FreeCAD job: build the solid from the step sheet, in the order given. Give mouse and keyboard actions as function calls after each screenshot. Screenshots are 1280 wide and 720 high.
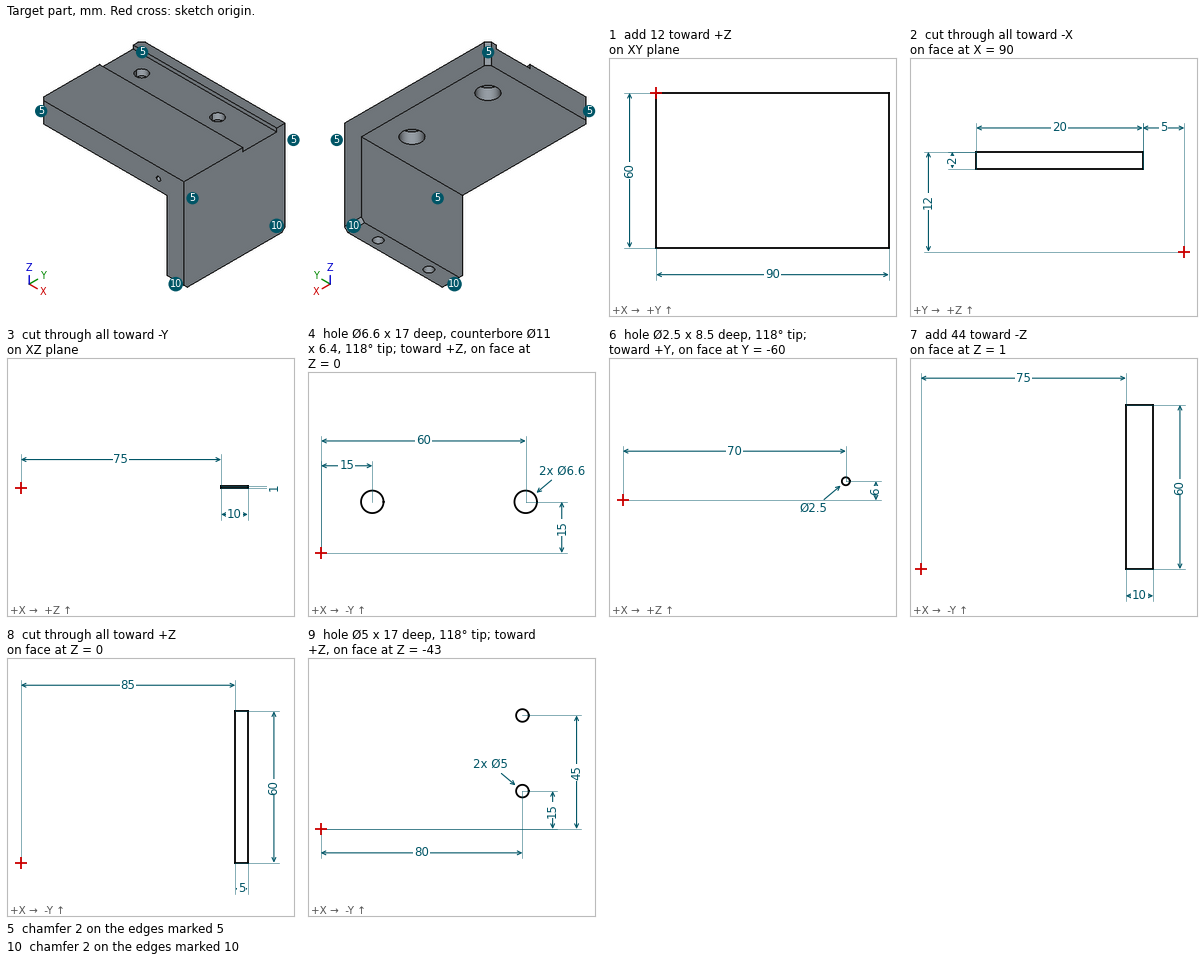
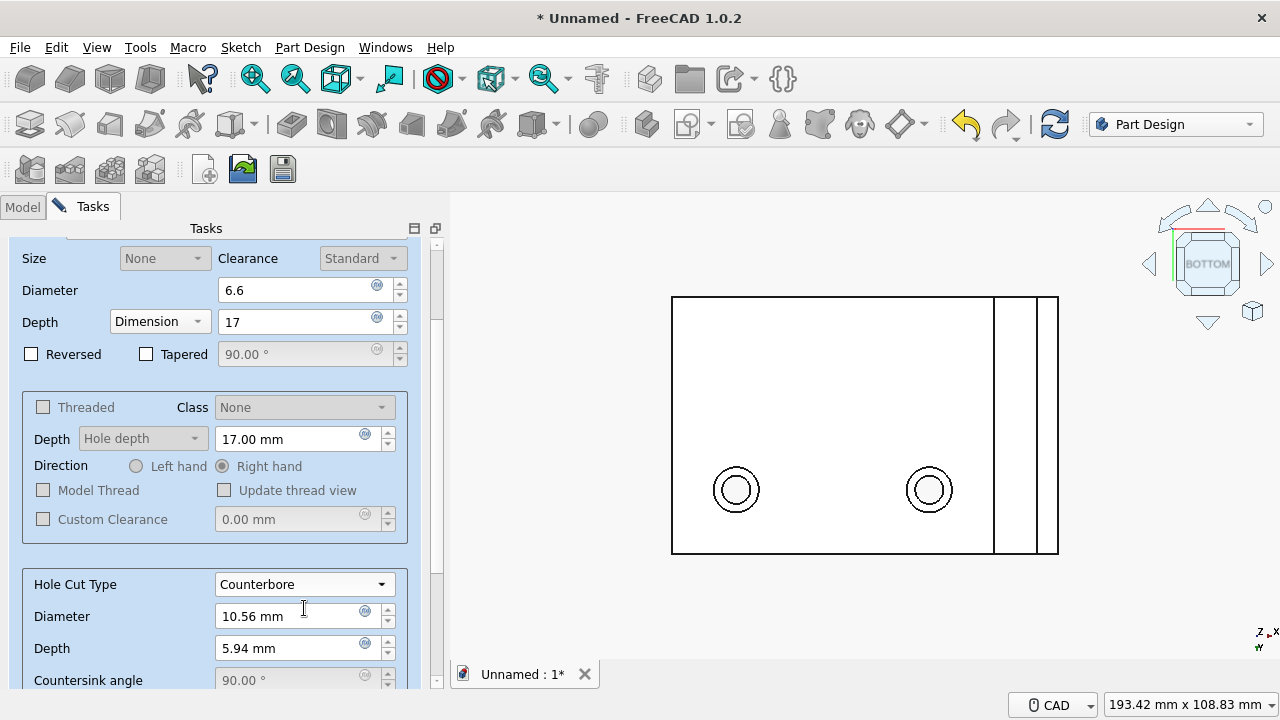
triple_click(298, 616)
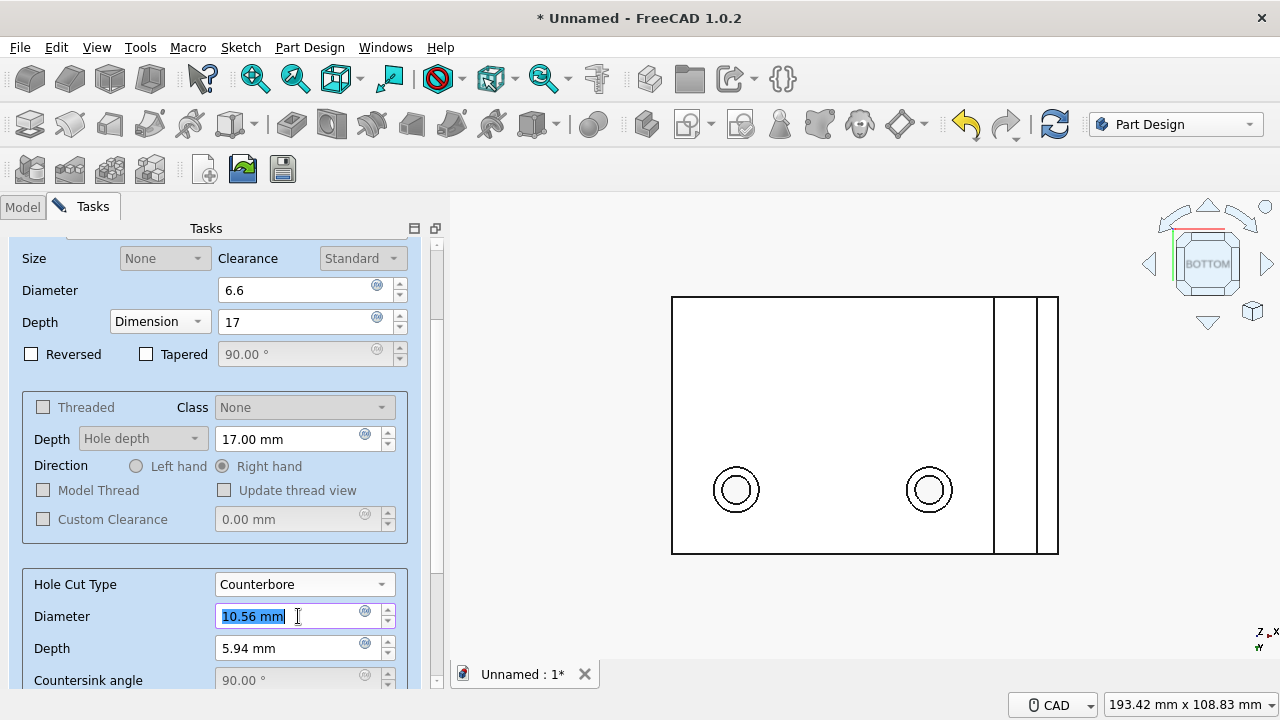
text(11)
key(Tab)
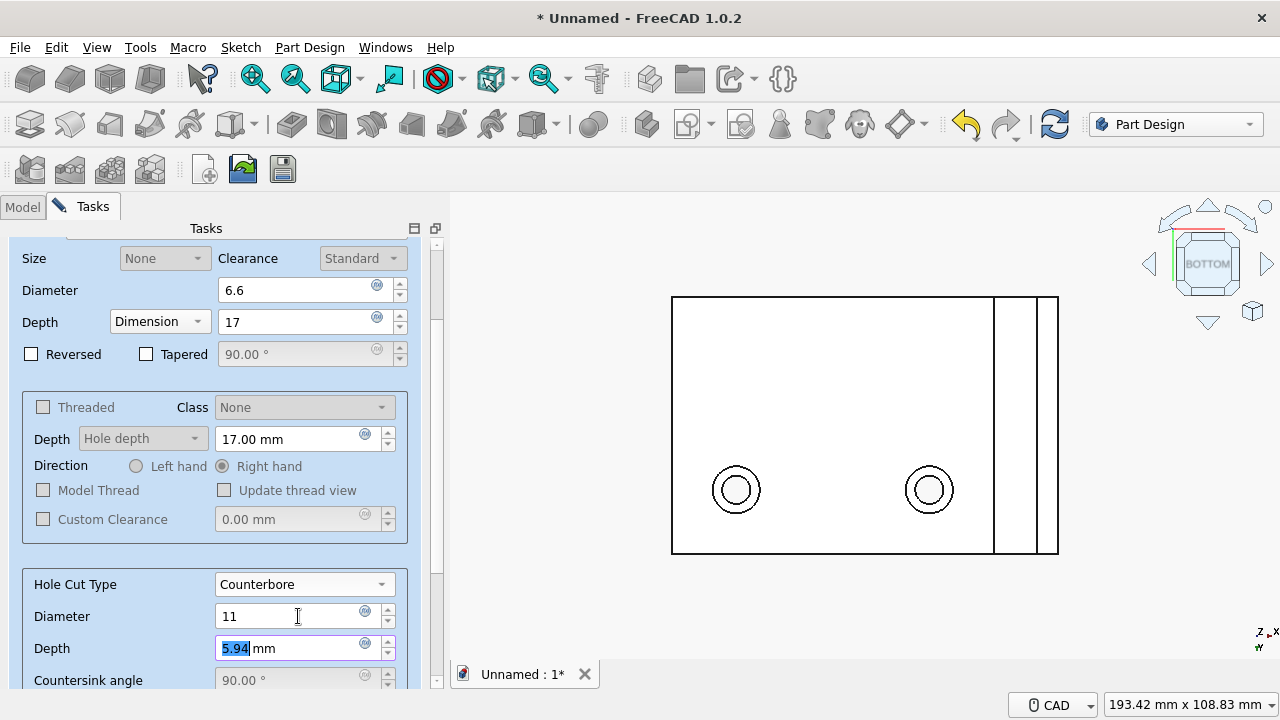
text(6.4)
key(Tab)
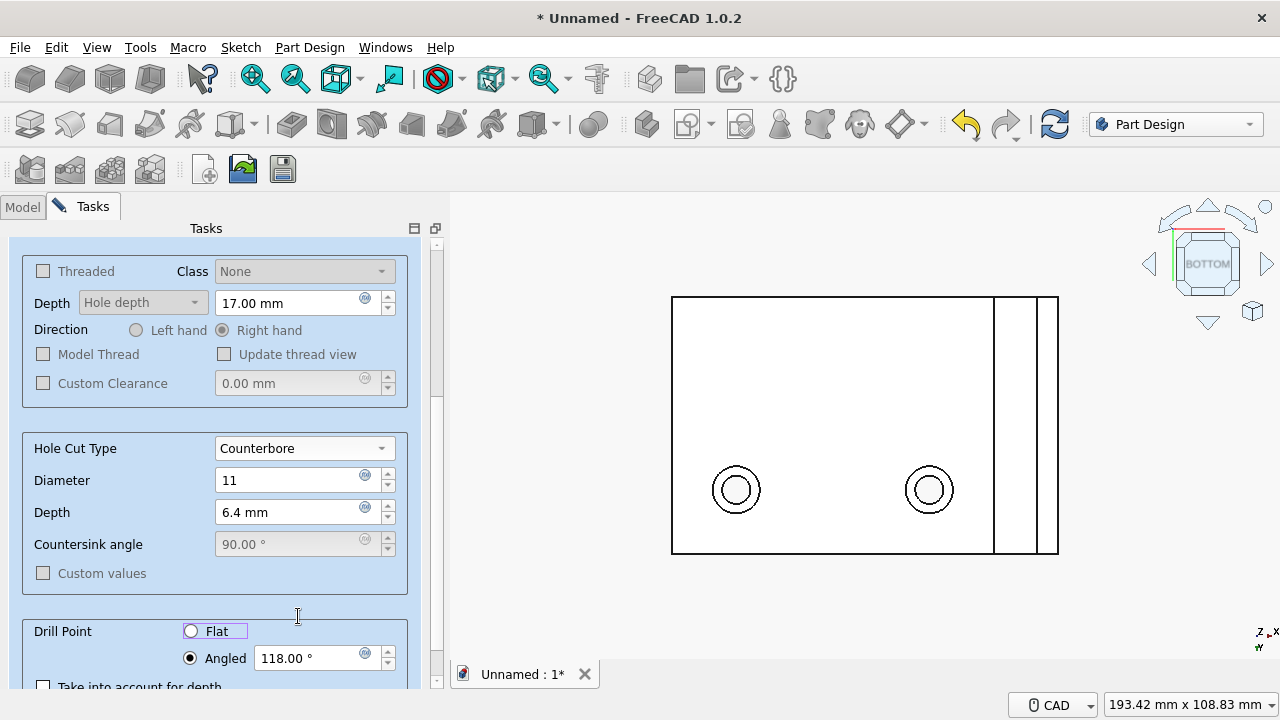
scroll(437, 463, up, 6)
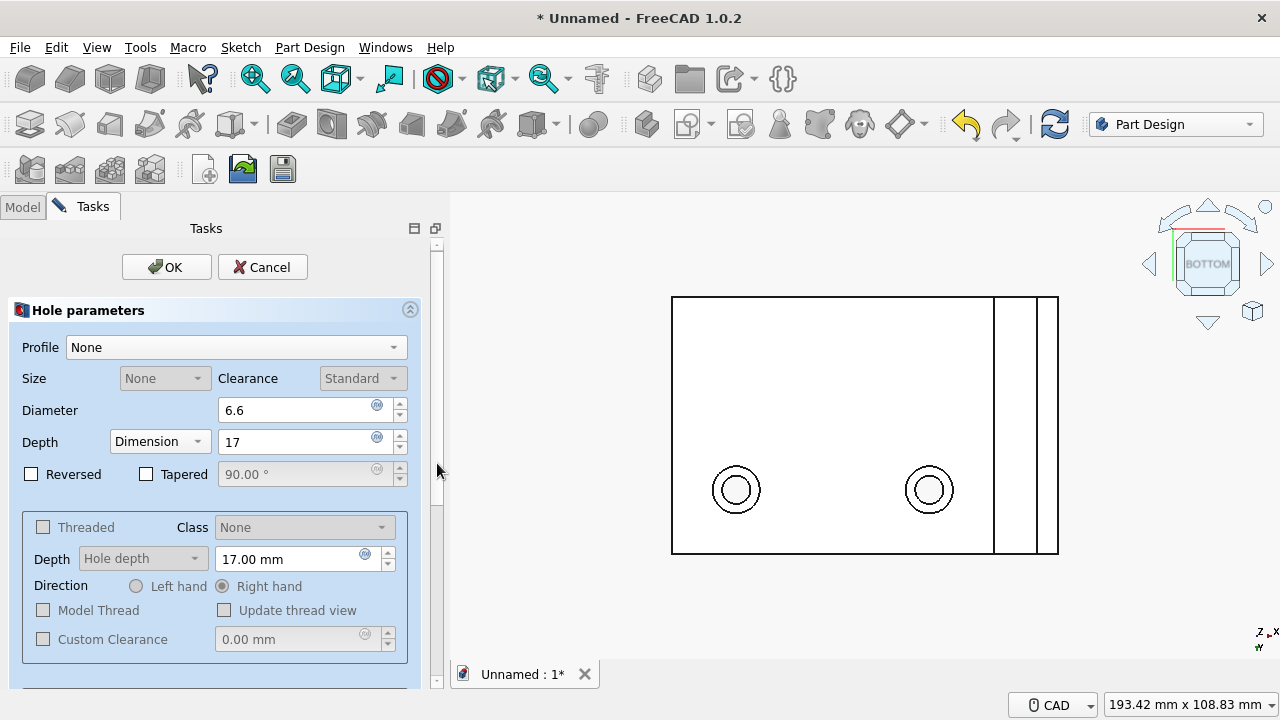
click(167, 267)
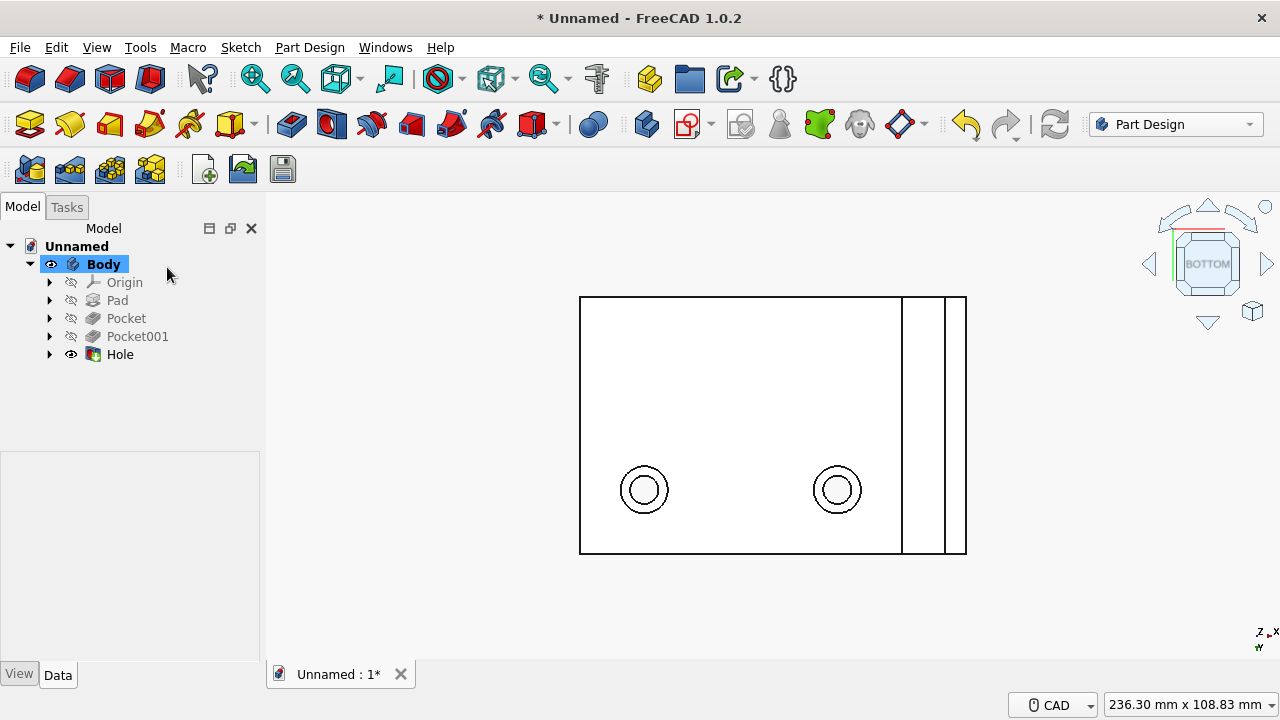
key(0)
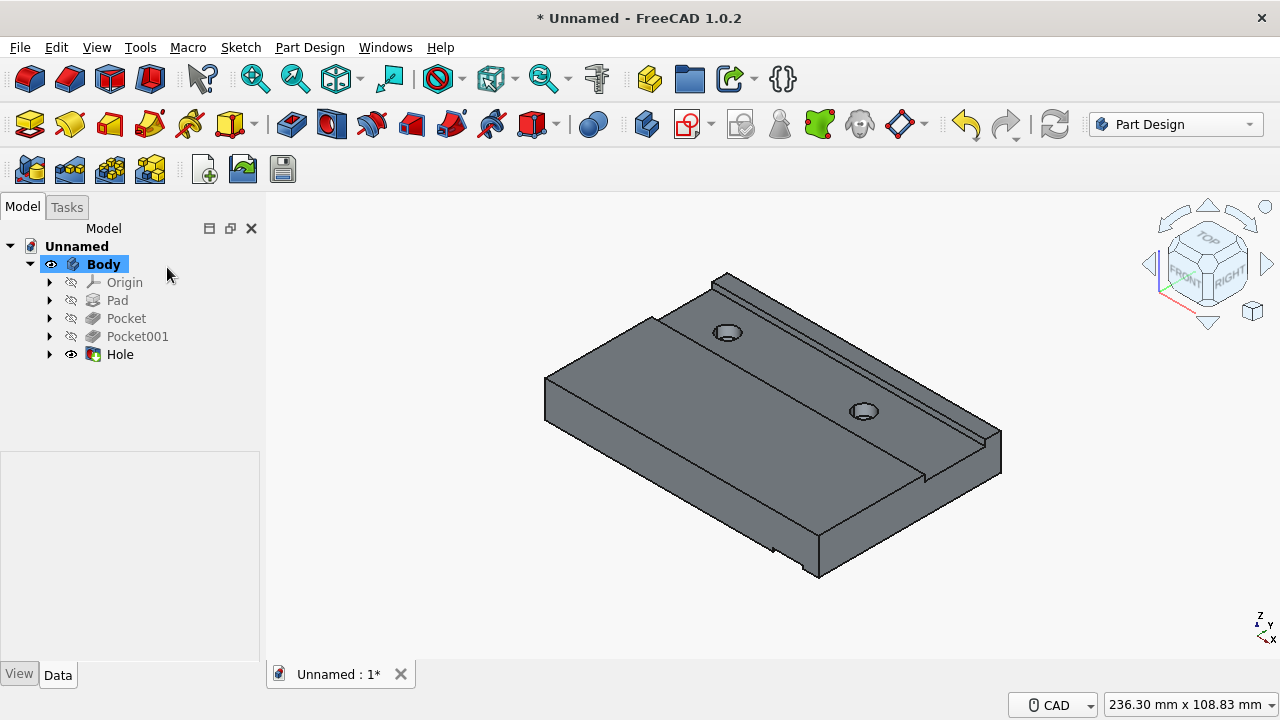
click(819, 556)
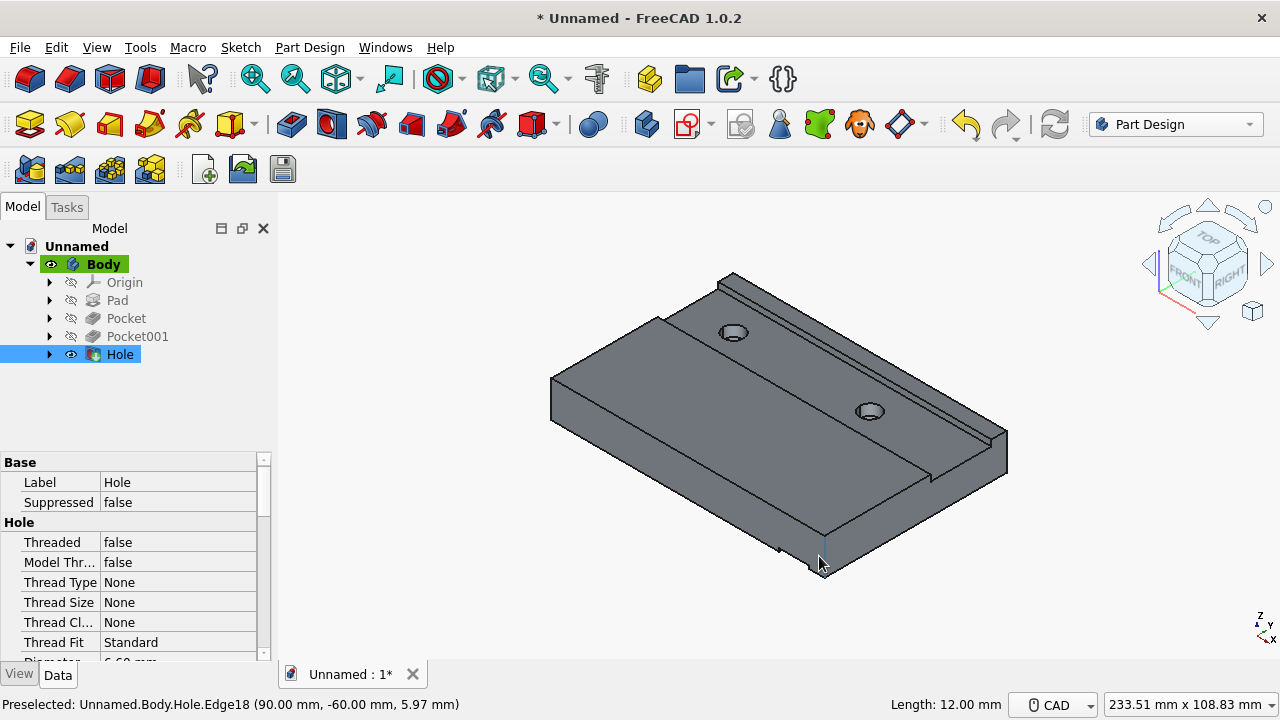
key(2)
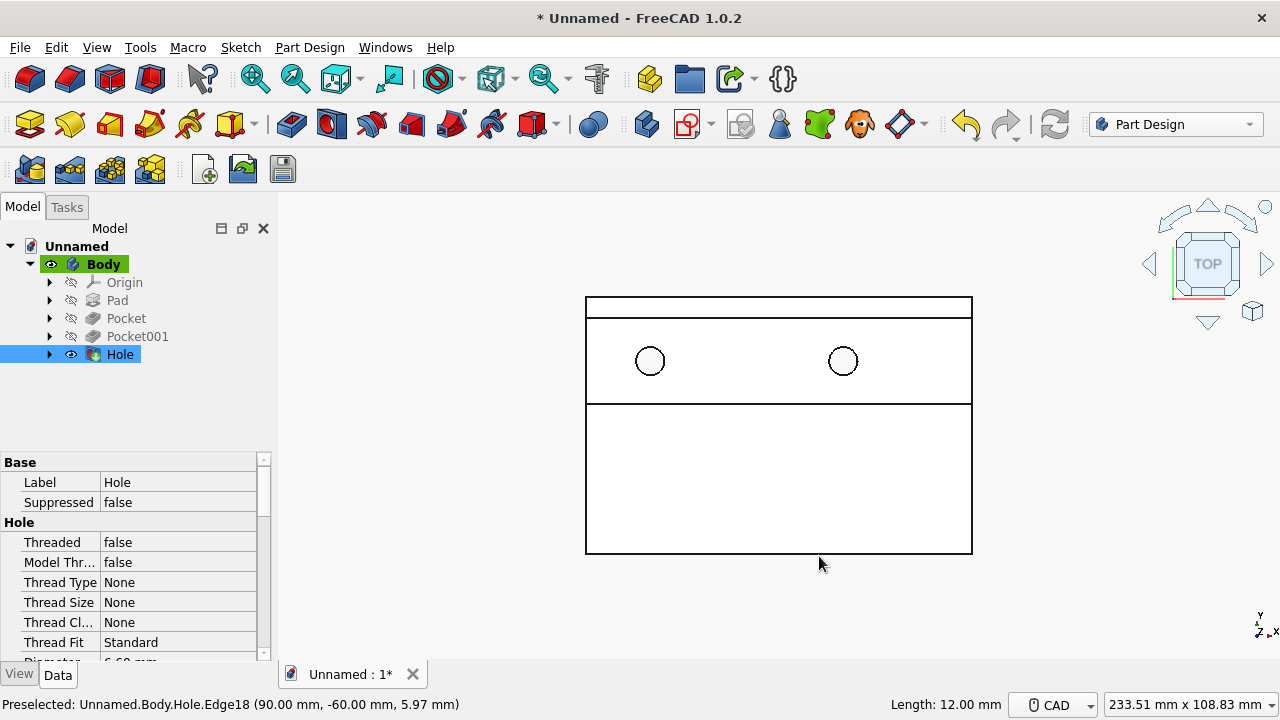
key(1)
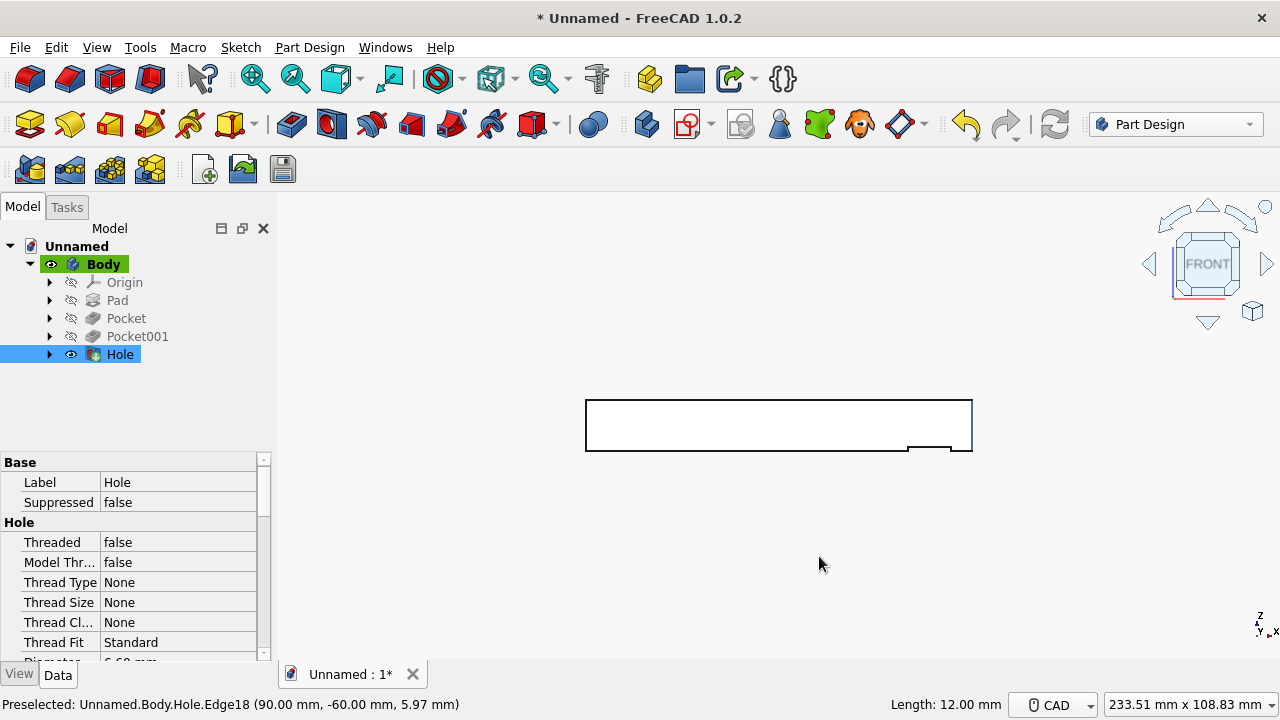
click(256, 80)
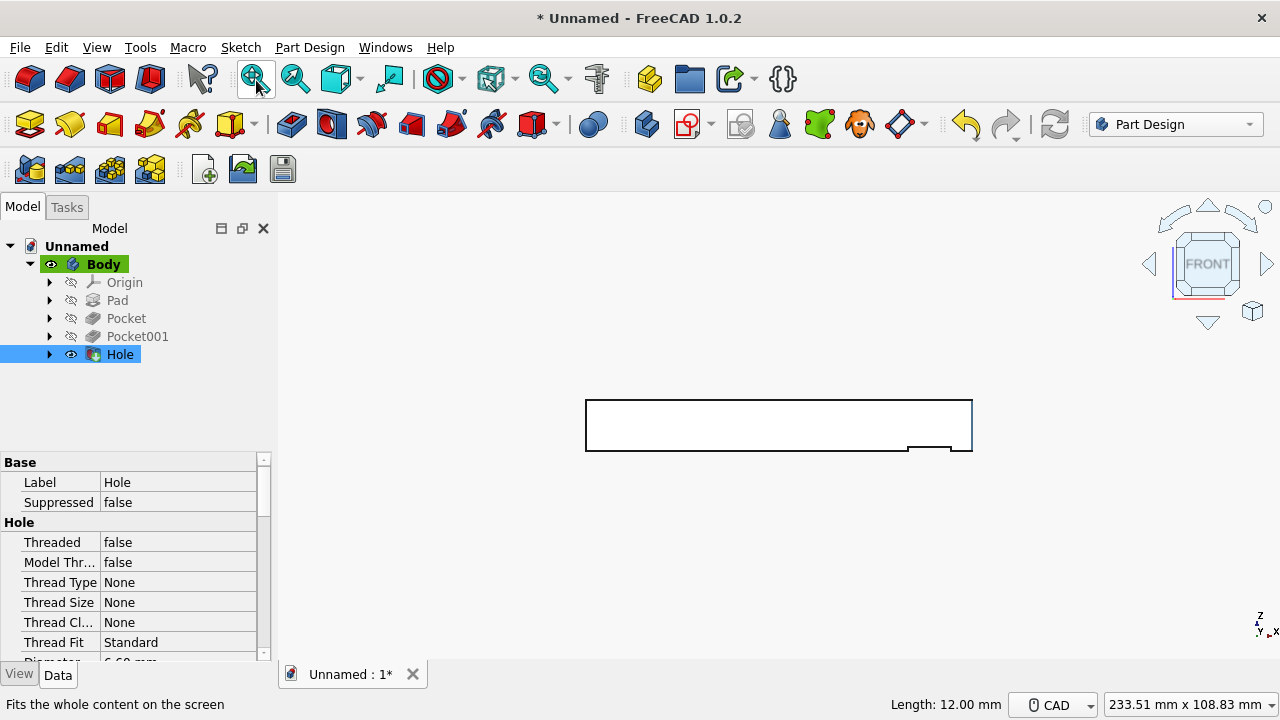
click(586, 425, ctrl)